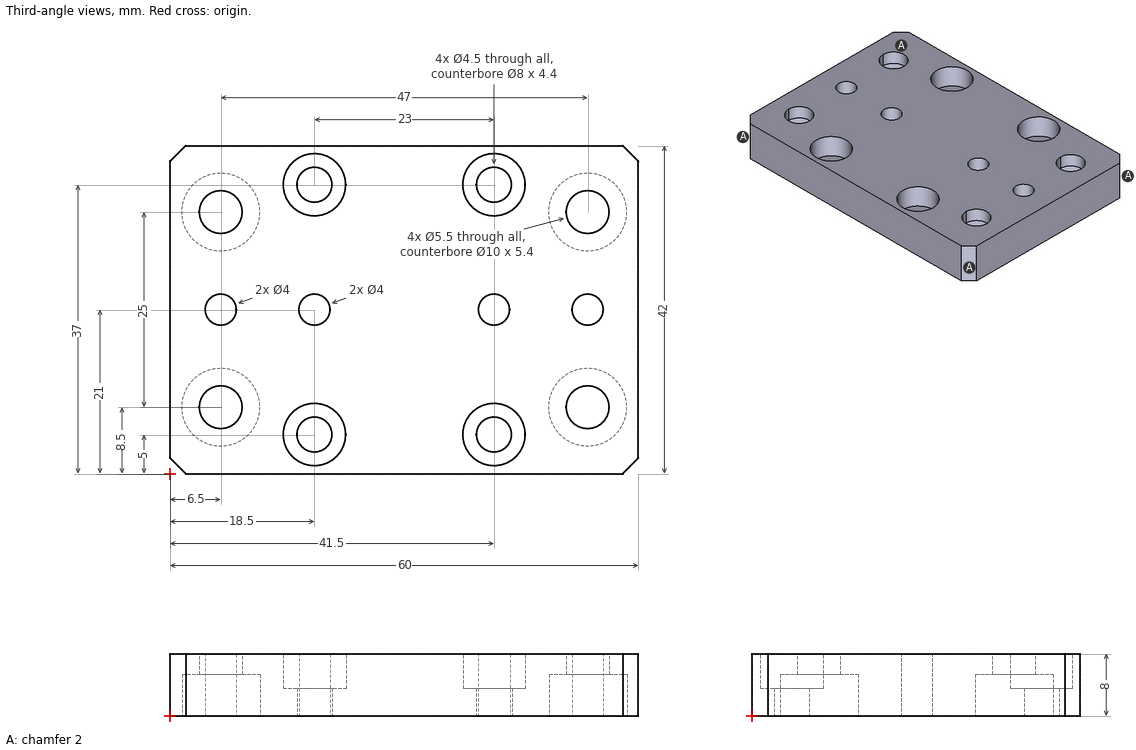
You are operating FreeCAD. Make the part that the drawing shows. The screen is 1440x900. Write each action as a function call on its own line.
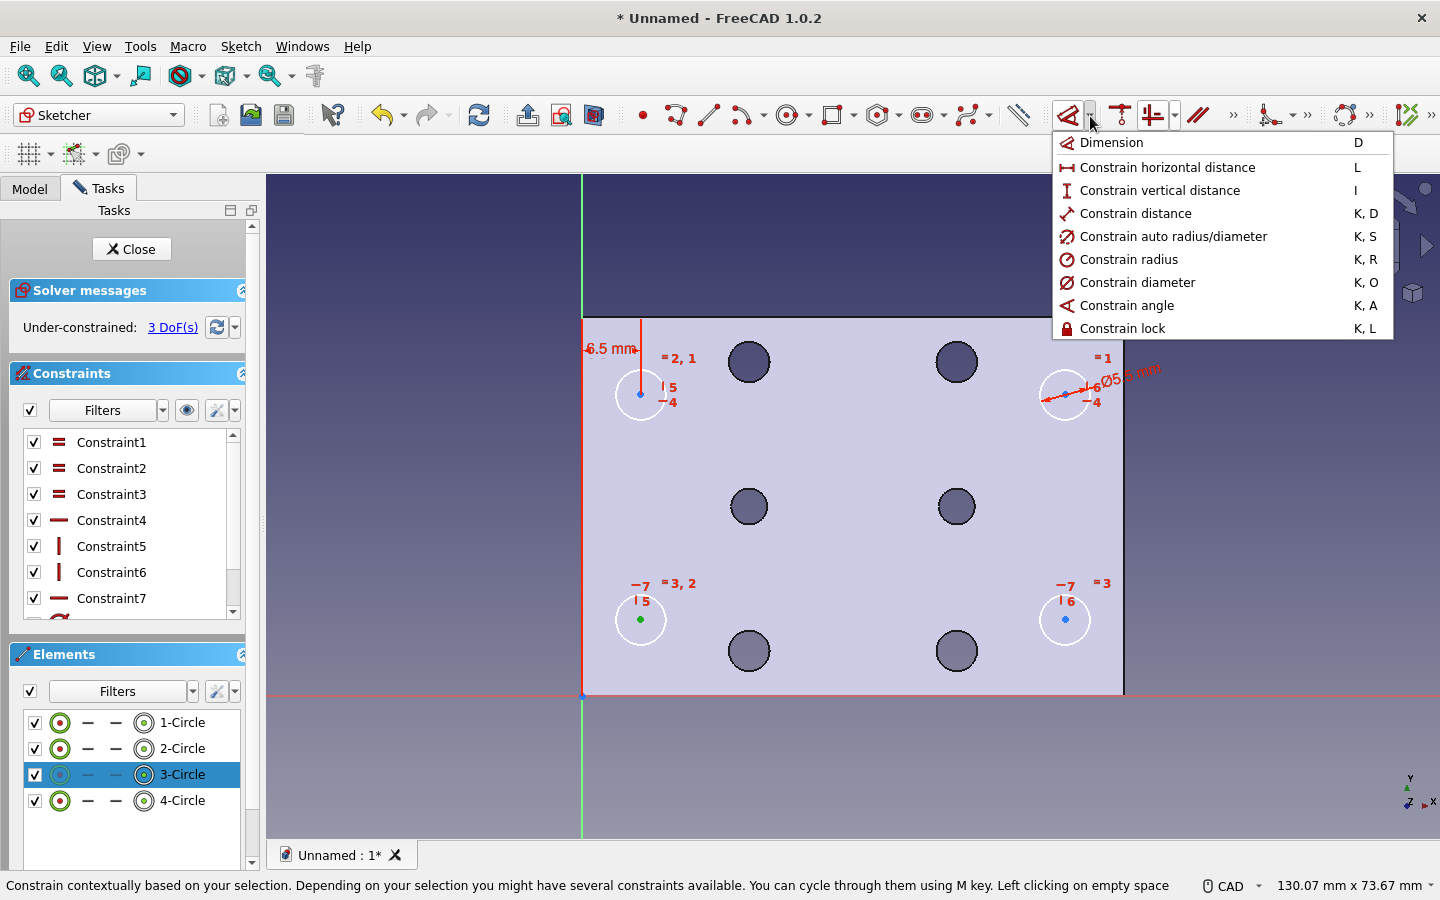
click(1223, 190)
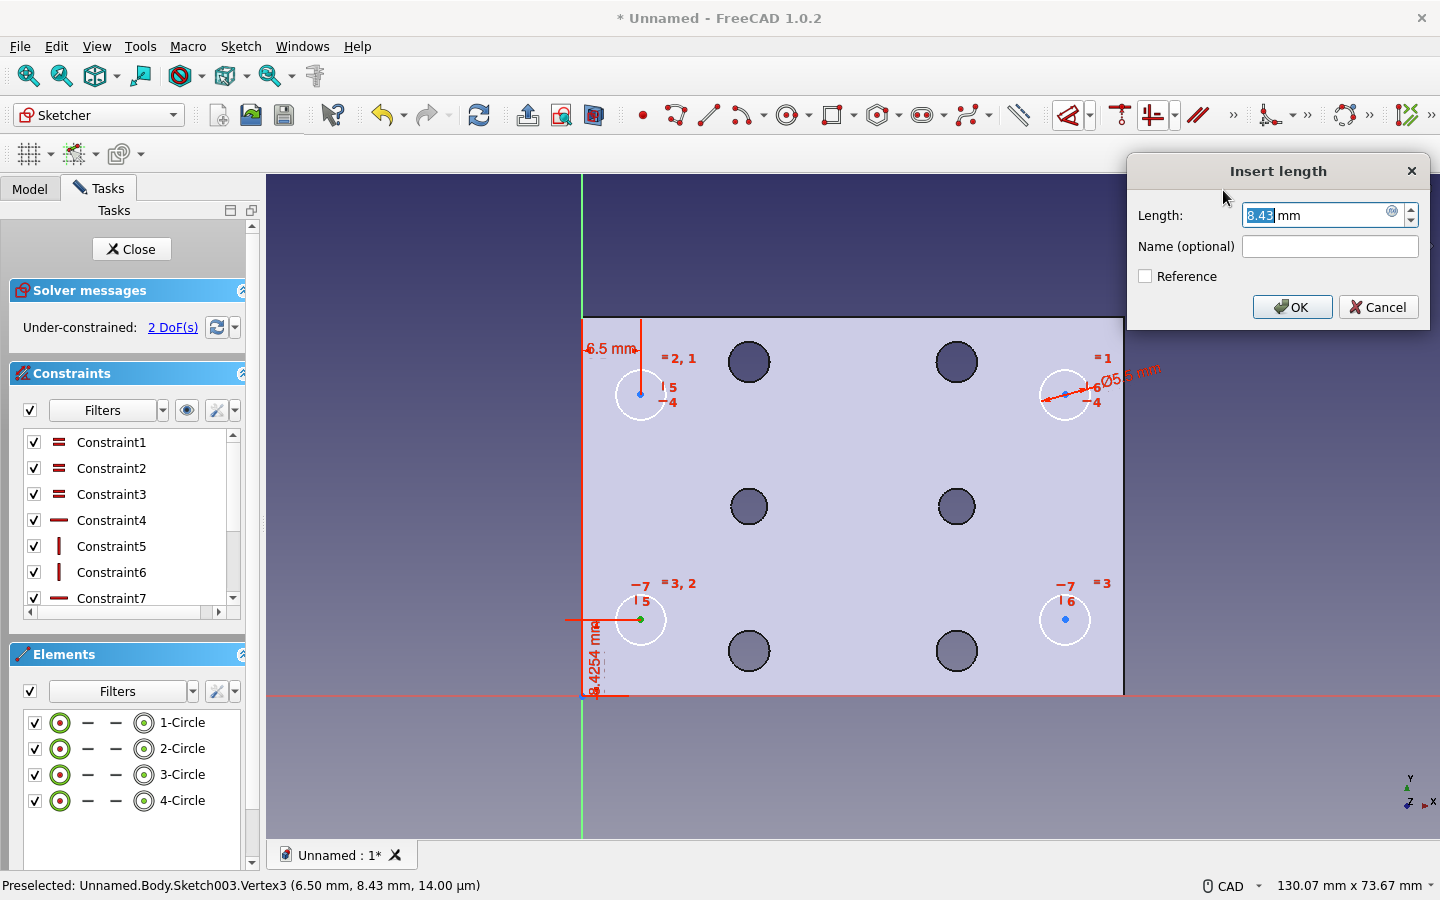
text(8.5)
key(Return)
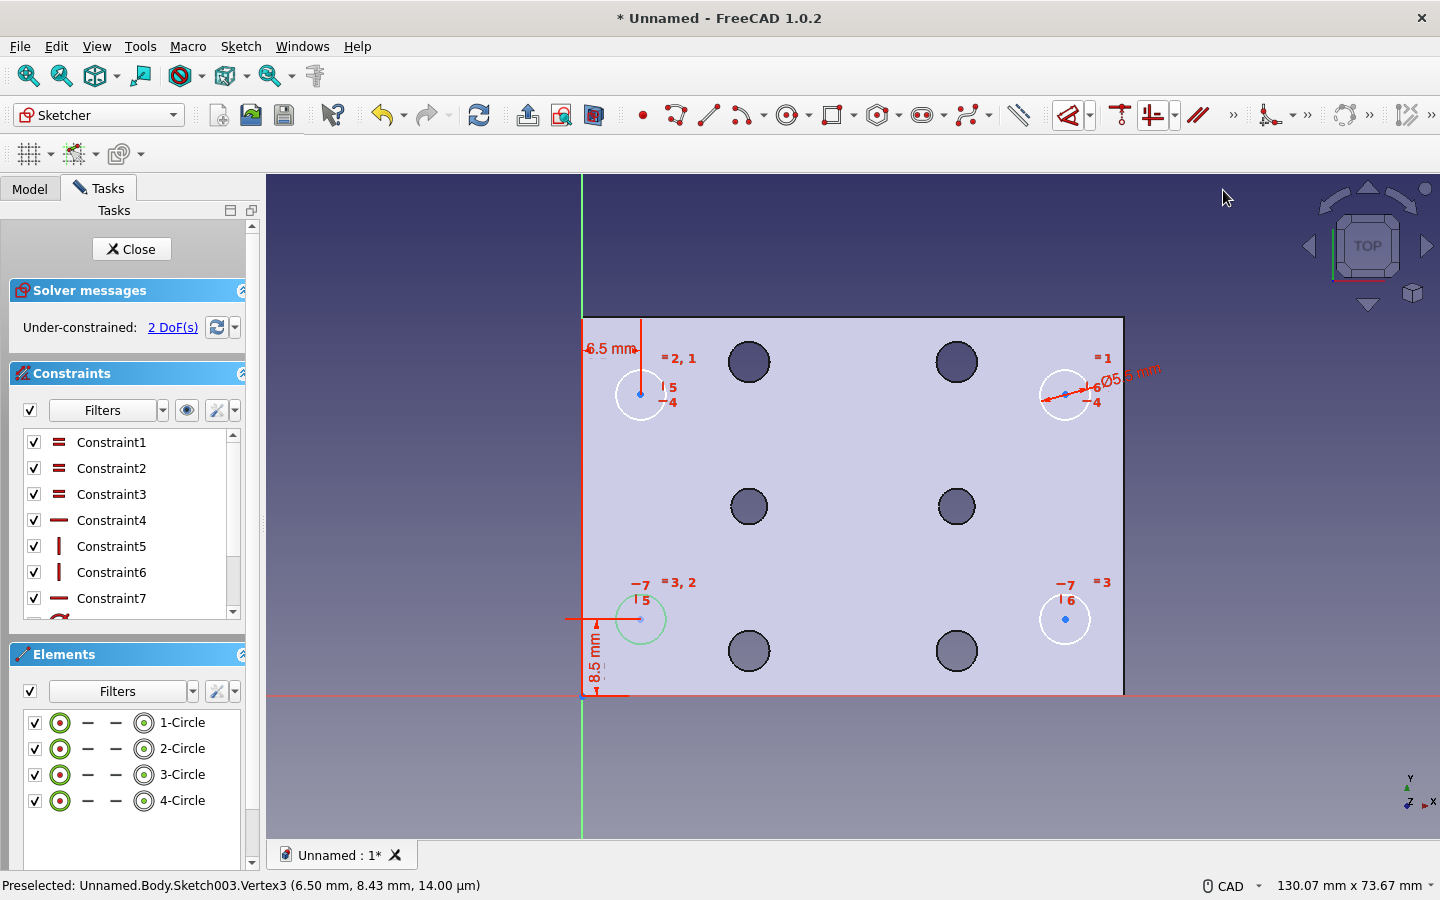
click(1065, 395)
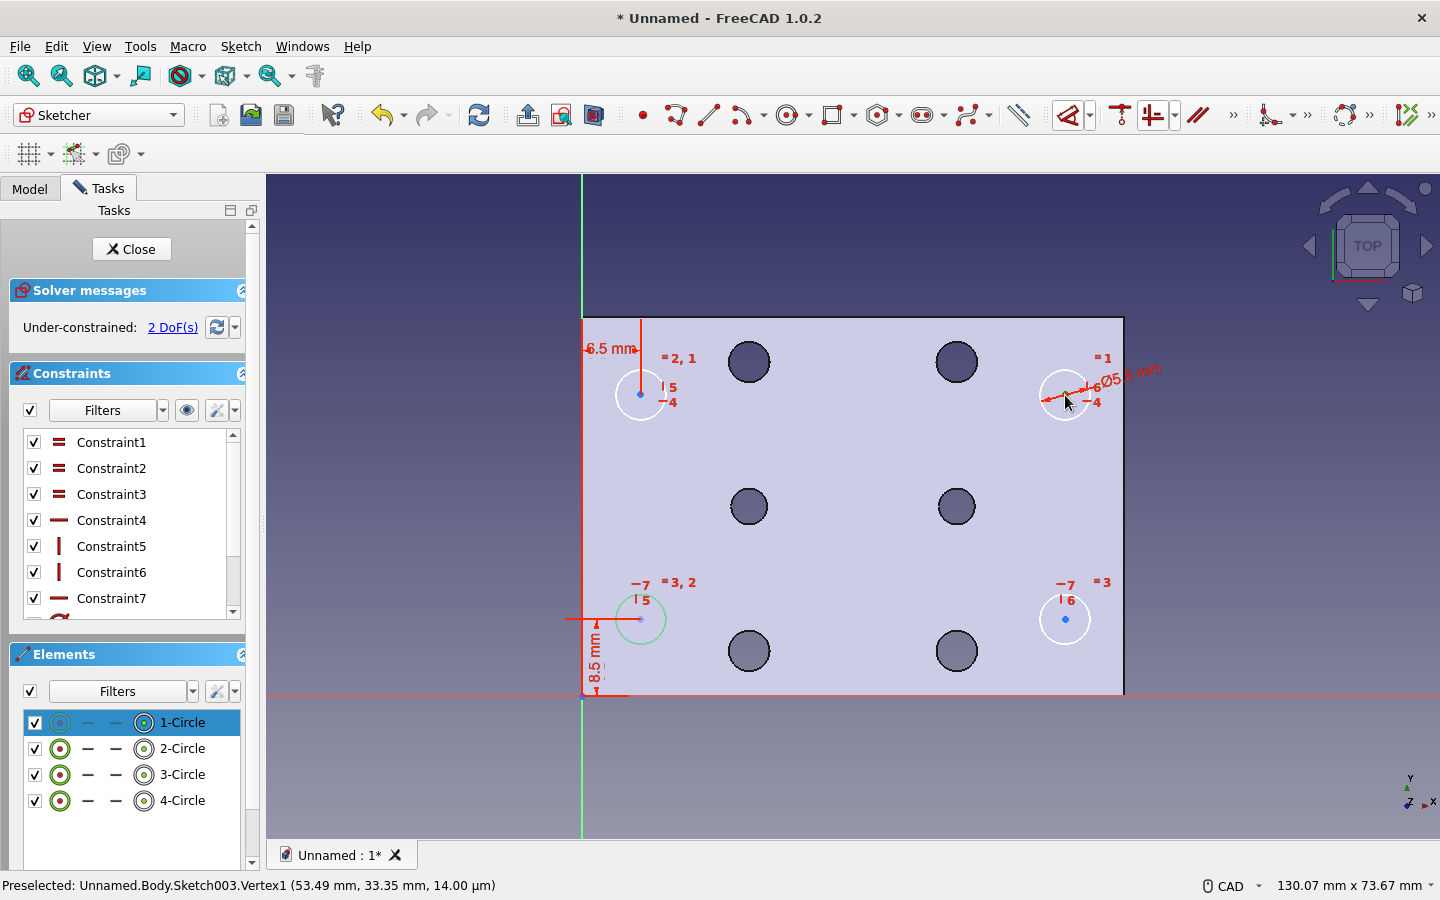
click(641, 395)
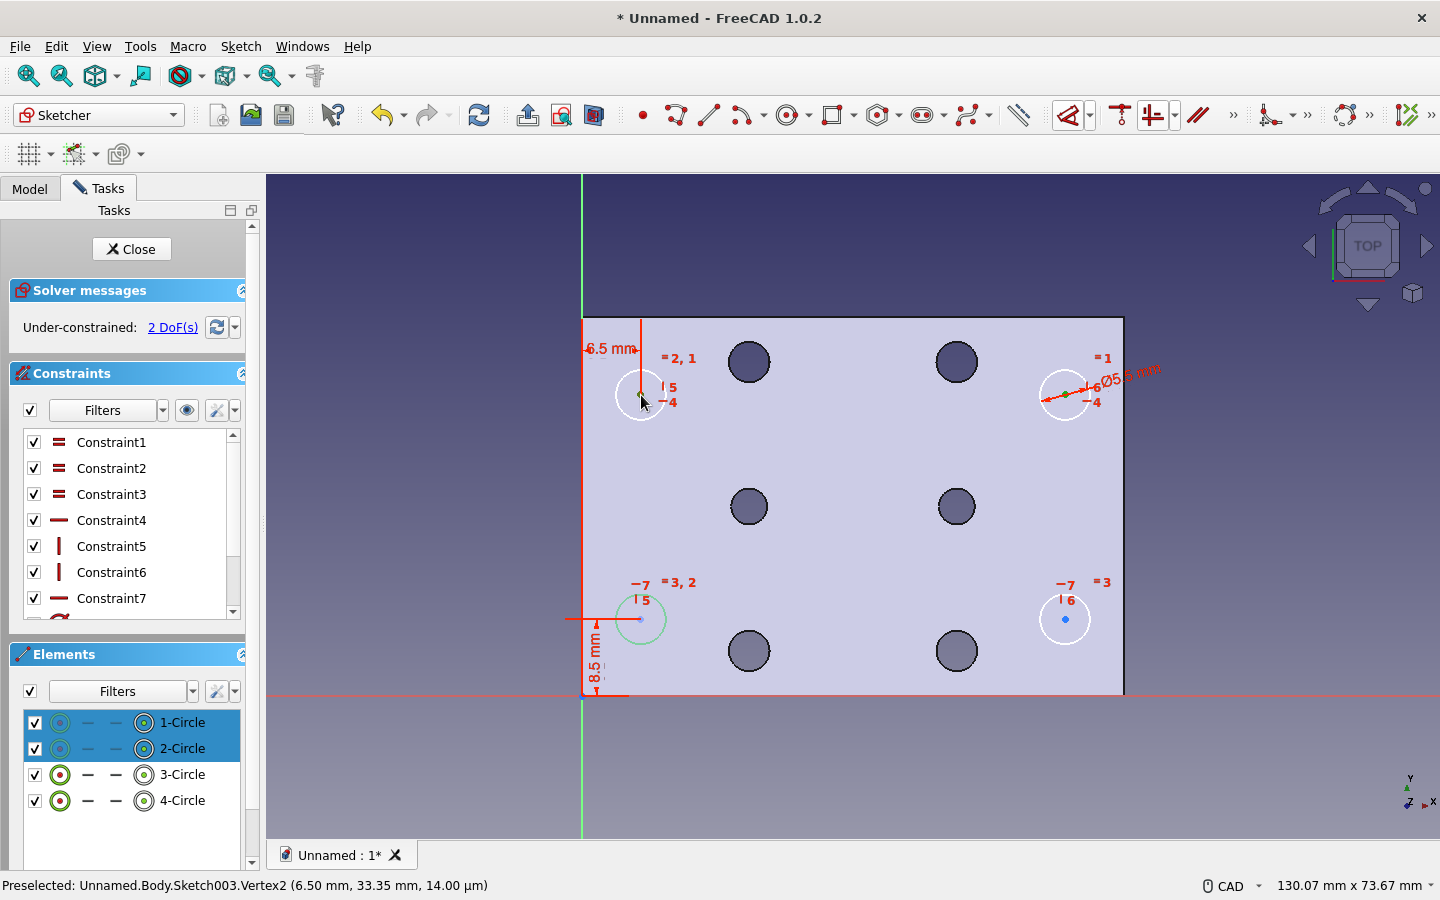
key(l)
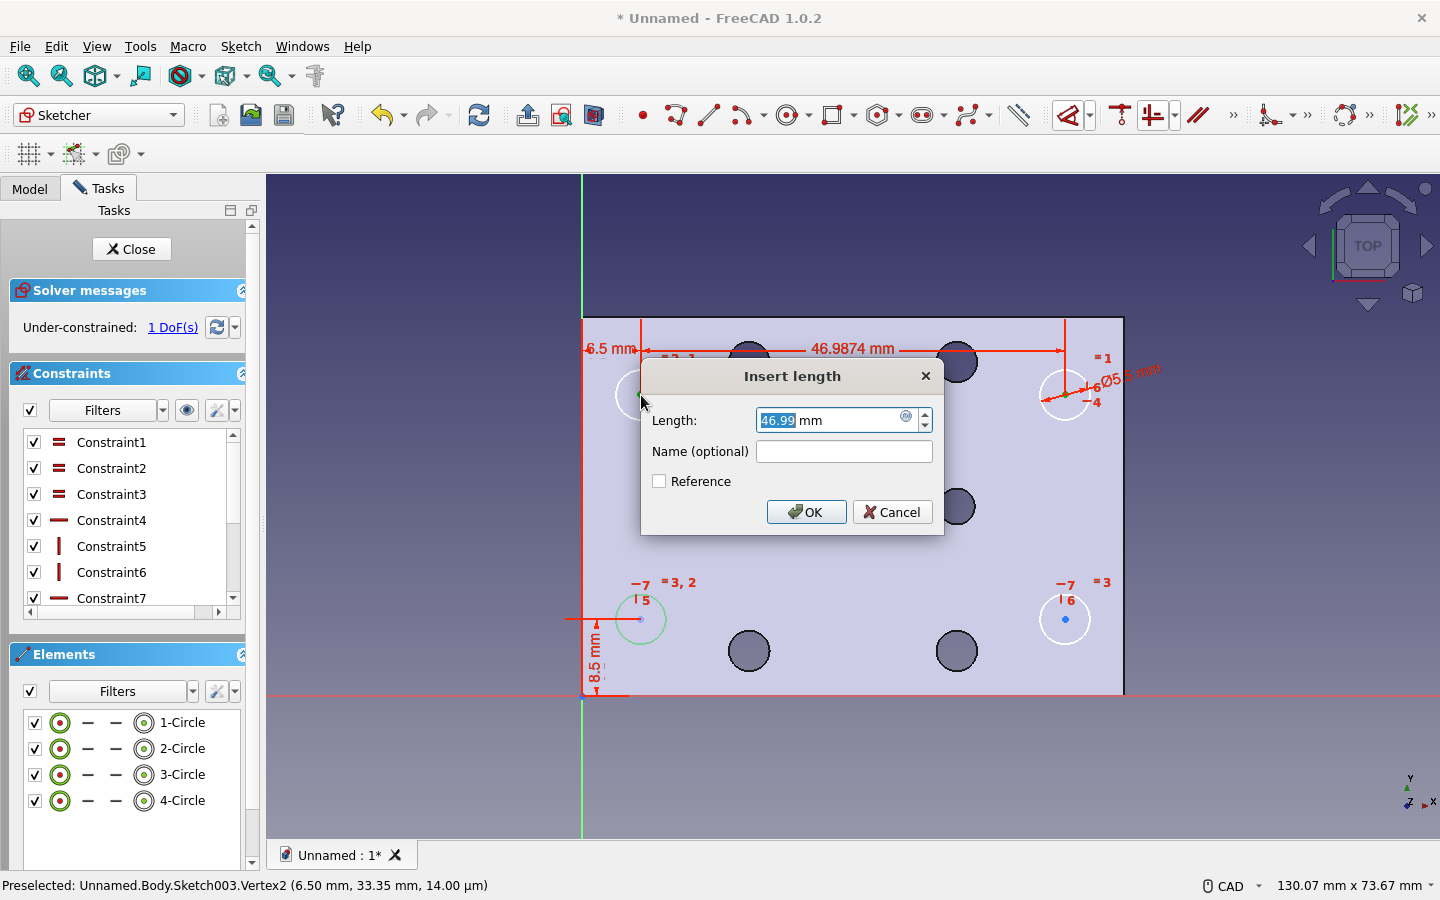
text(47)
key(Return)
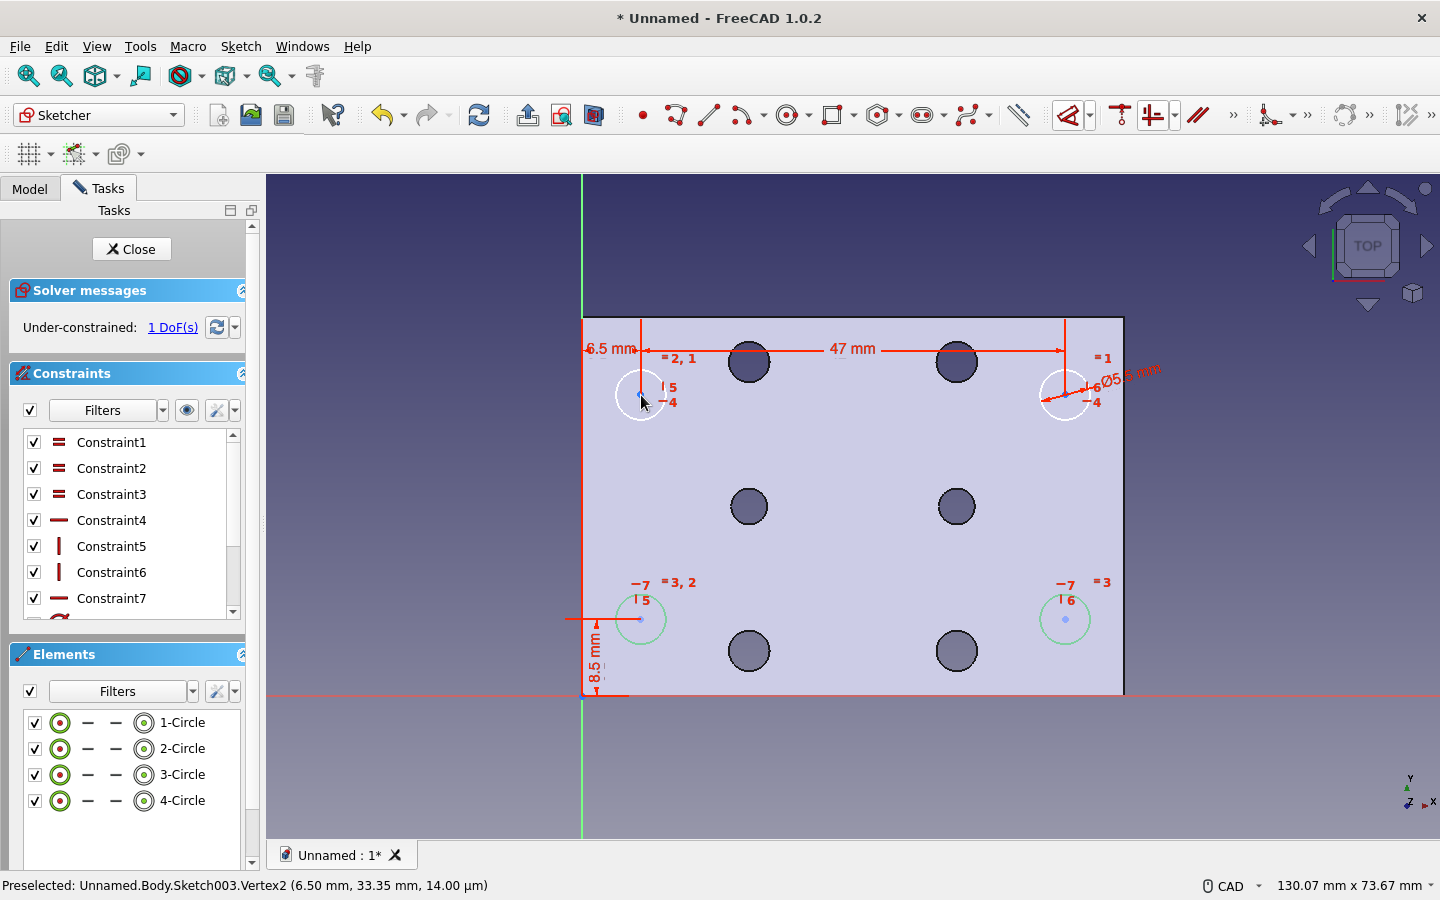
click(641, 395)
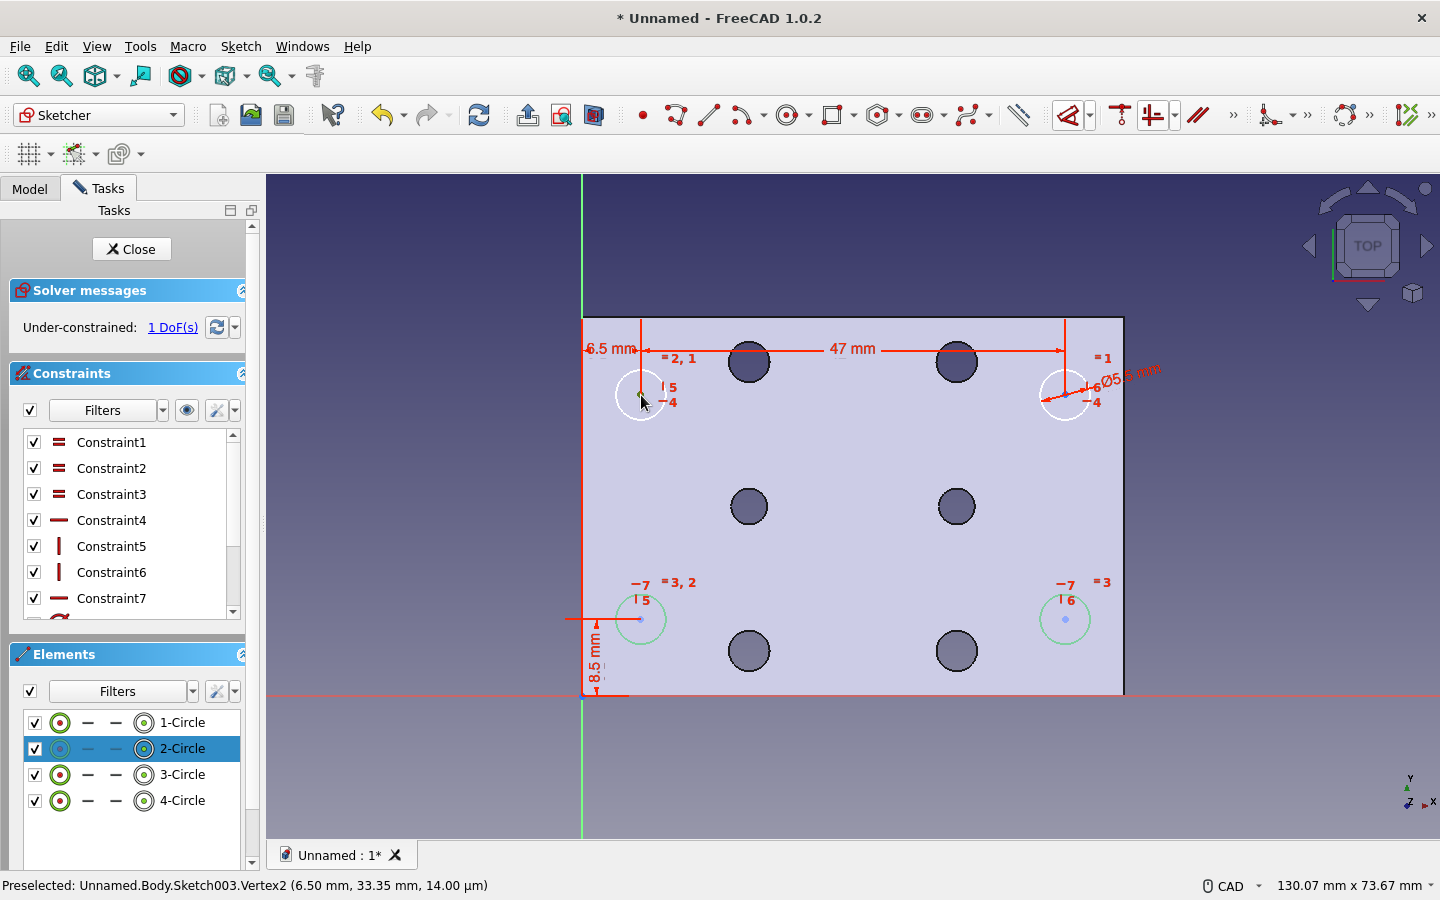
click(641, 619)